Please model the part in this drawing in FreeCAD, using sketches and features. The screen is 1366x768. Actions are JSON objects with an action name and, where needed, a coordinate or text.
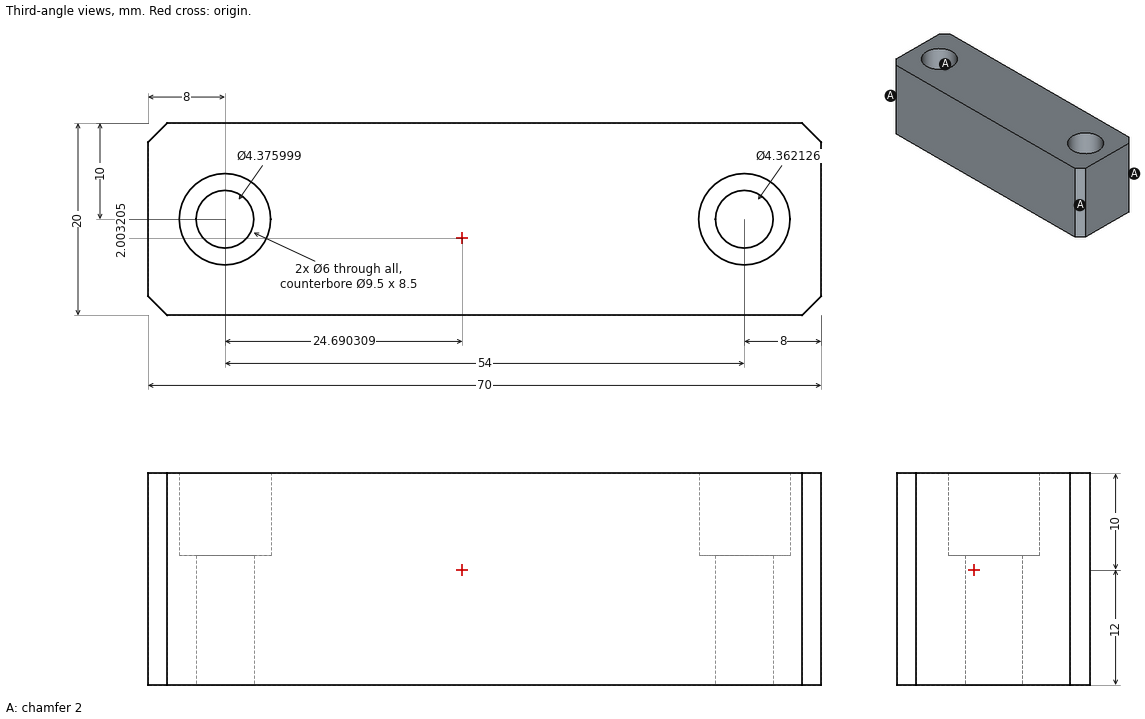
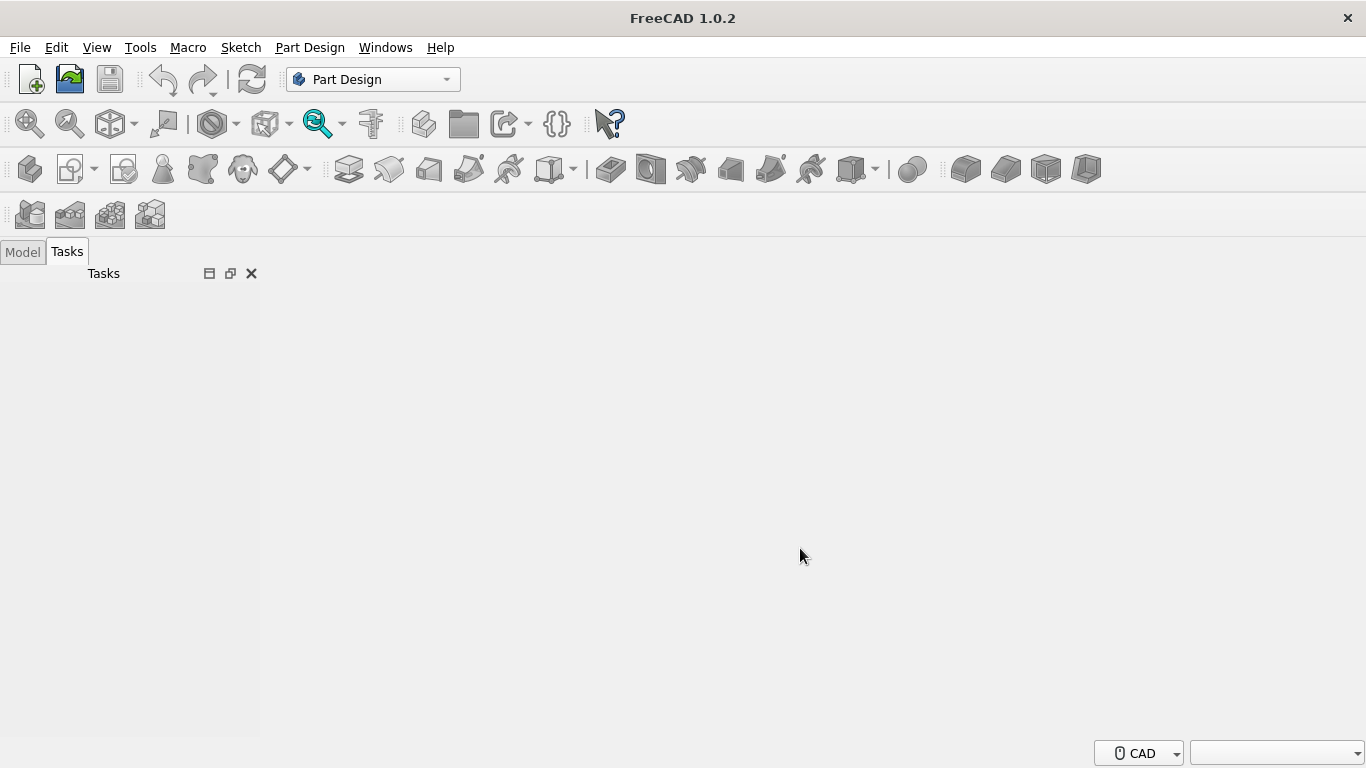
{"action": "left_click", "coordinate": [30, 80]}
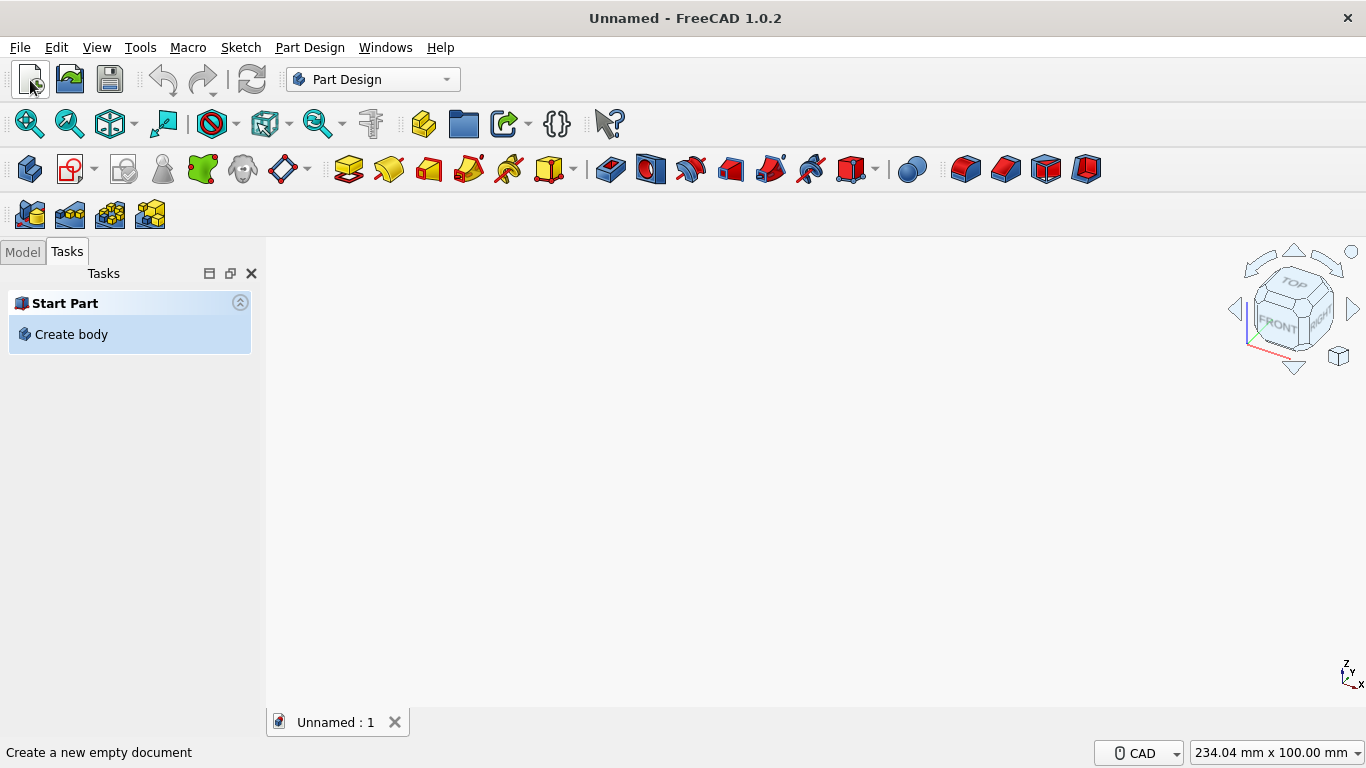
{"action": "left_click", "coordinate": [70, 170]}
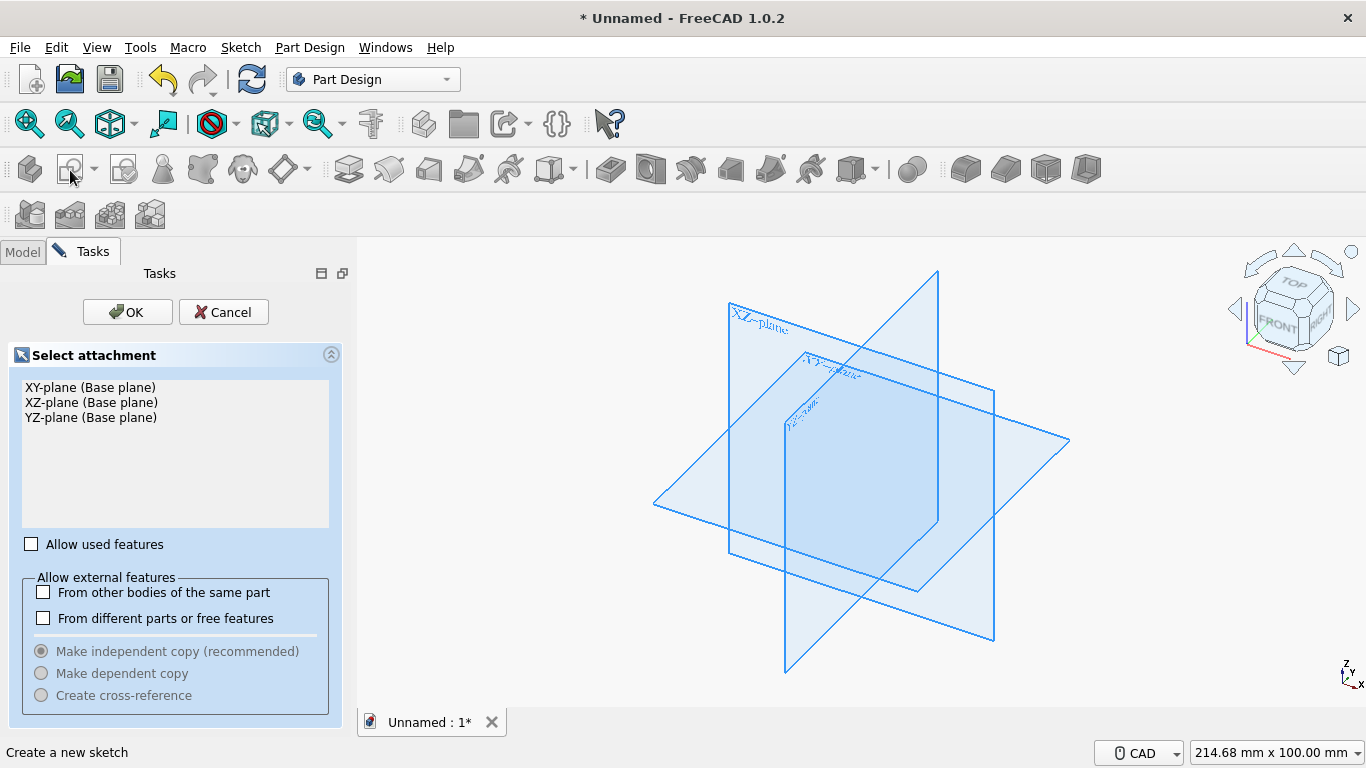
{"action": "left_click", "coordinate": [82, 388]}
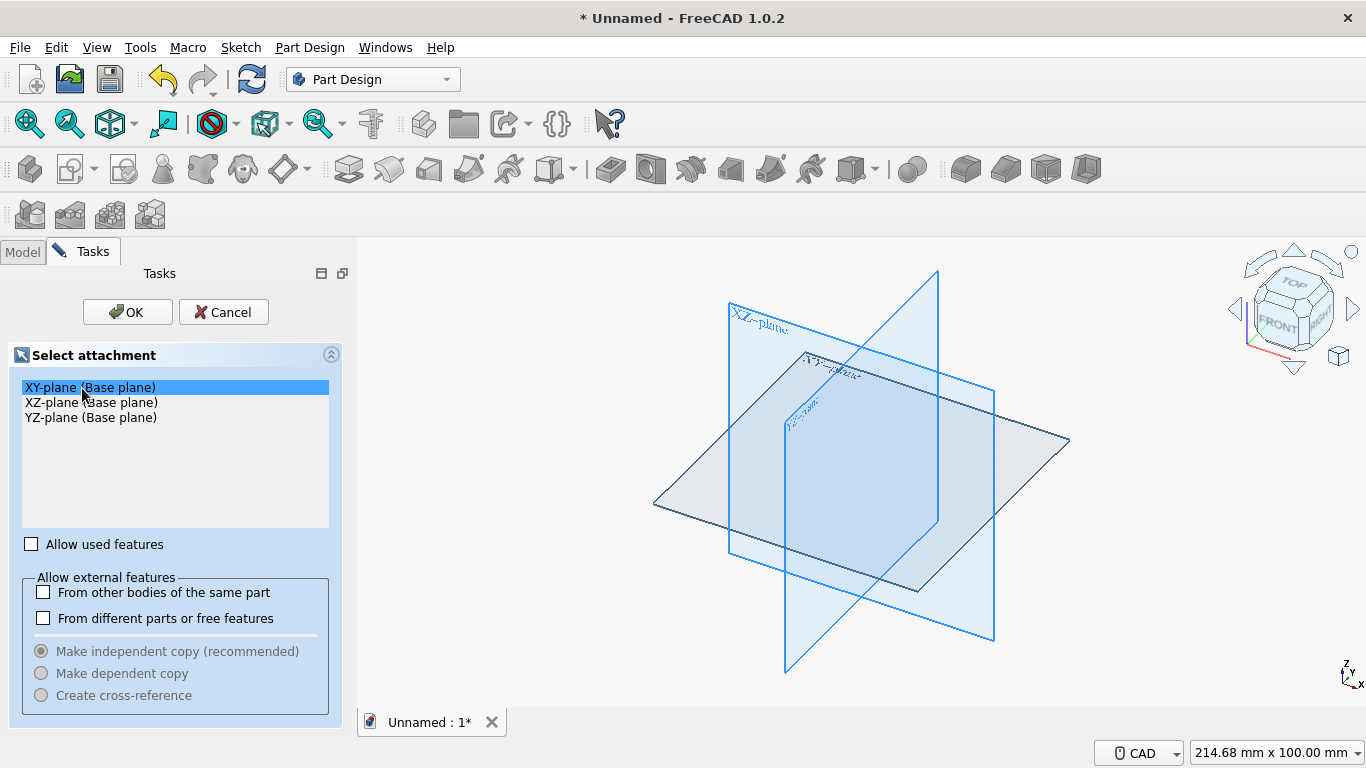
{"action": "left_click", "coordinate": [128, 312]}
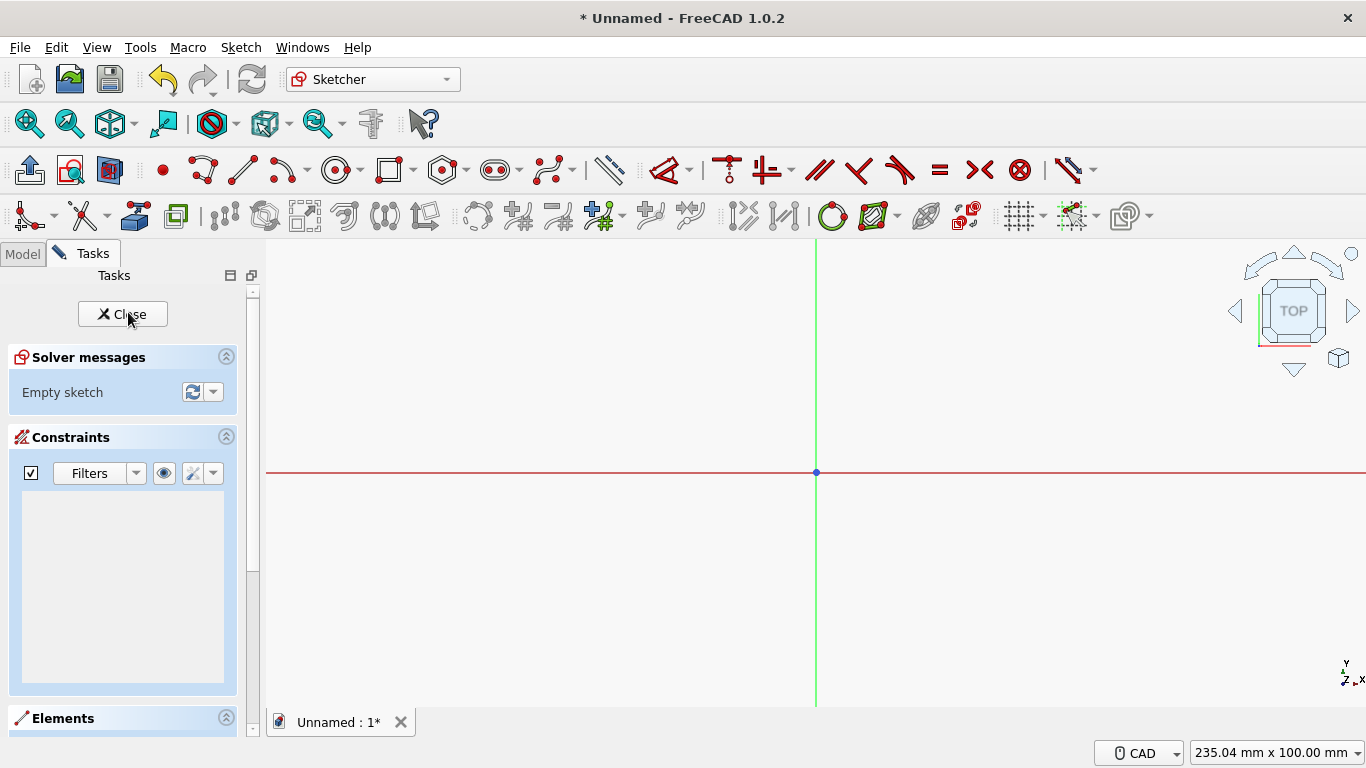
{"action": "scroll", "coordinate": [923, 452], "scroll_direction": "up", "scroll_amount": 3}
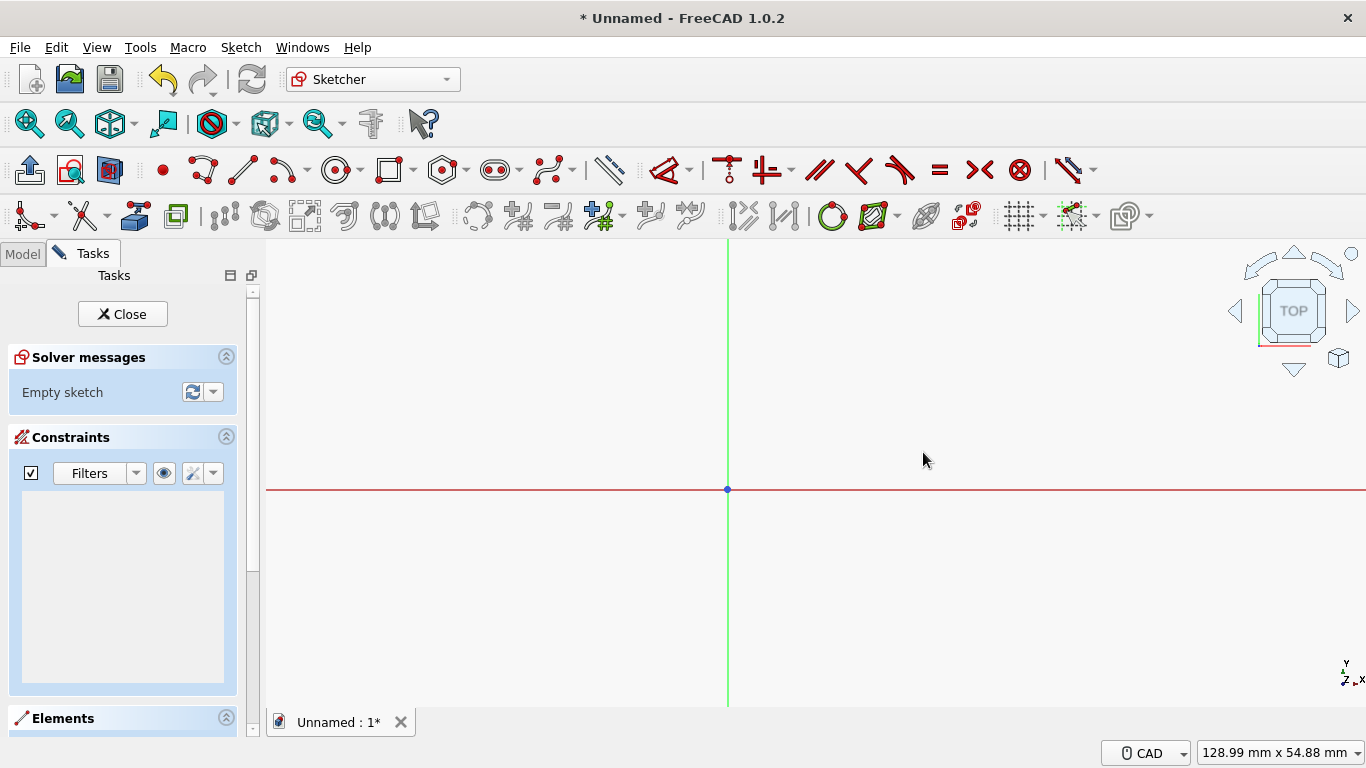
{"action": "left_click", "coordinate": [390, 170]}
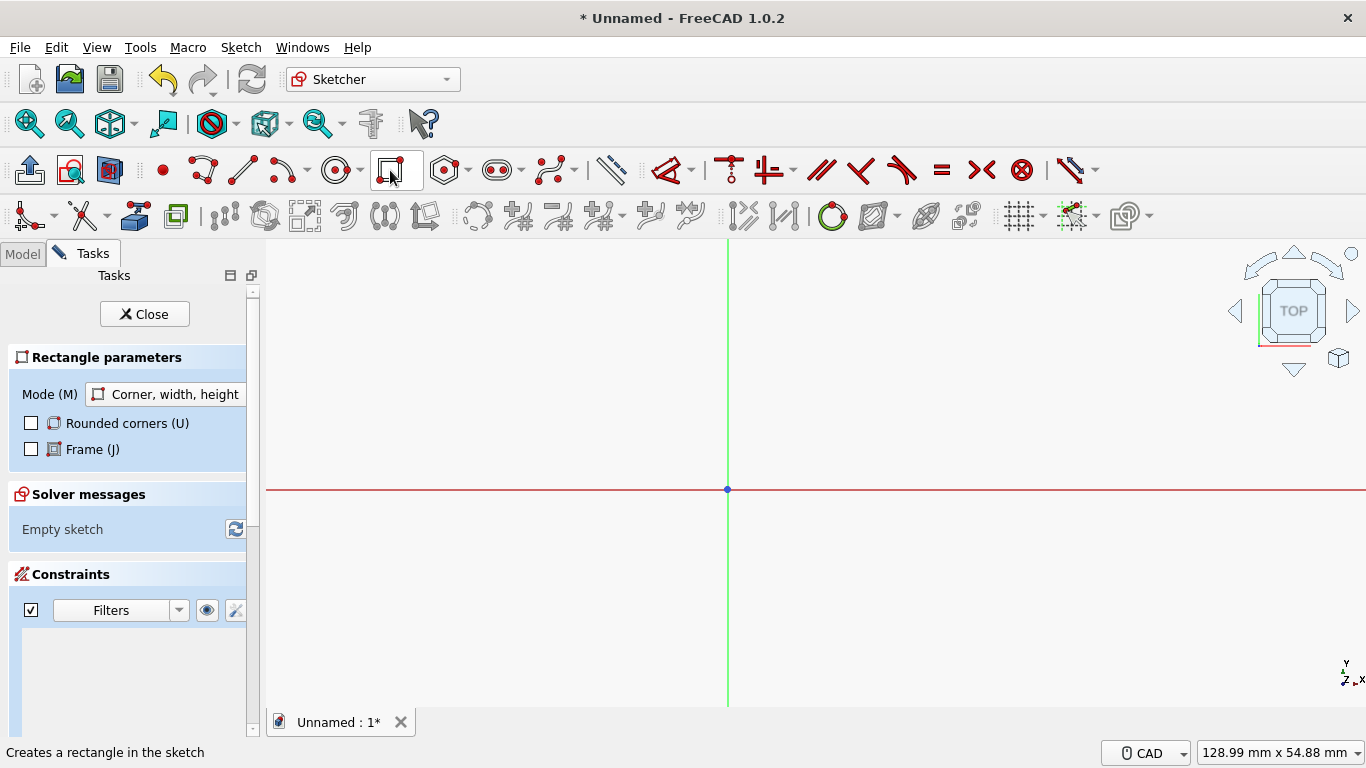
{"action": "left_click", "coordinate": [449, 388]}
{"action": "left_click", "coordinate": [1046, 558]}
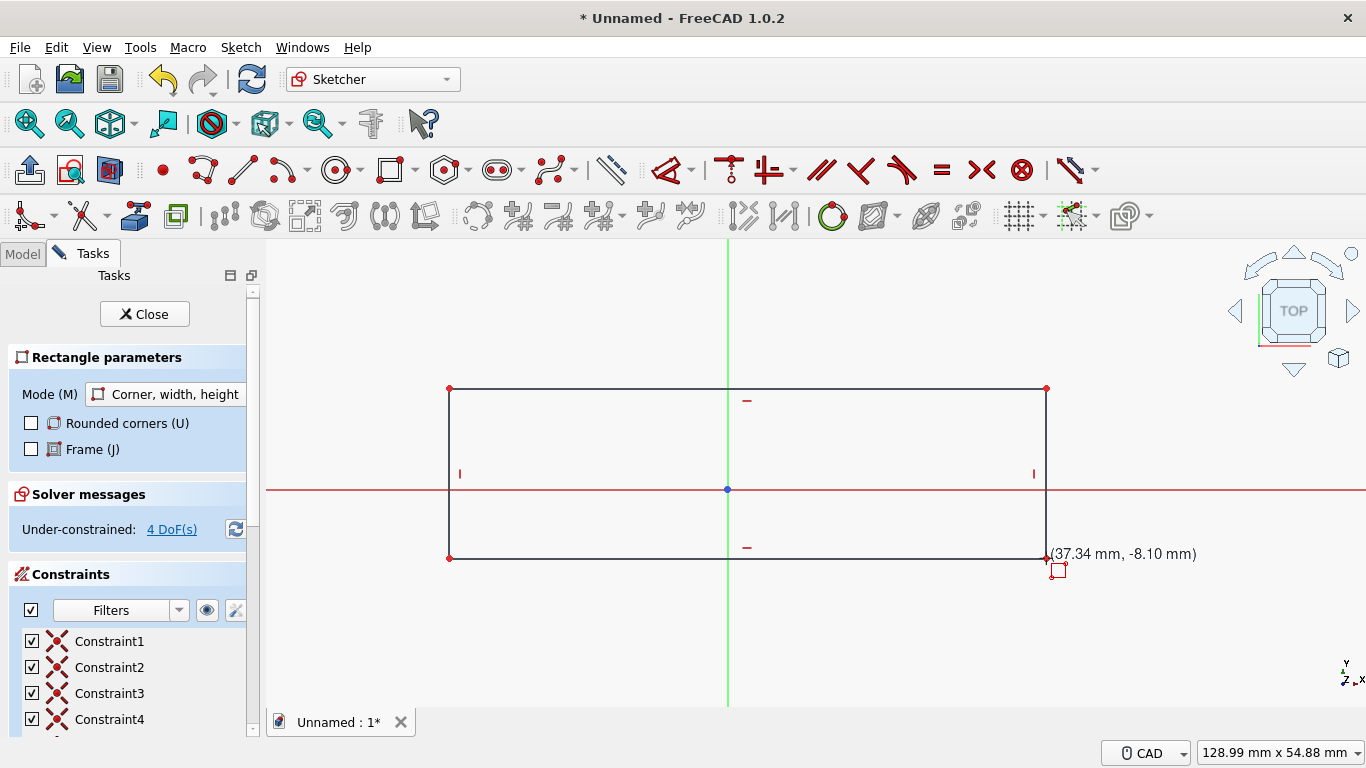
{"action": "key", "text": "g c"}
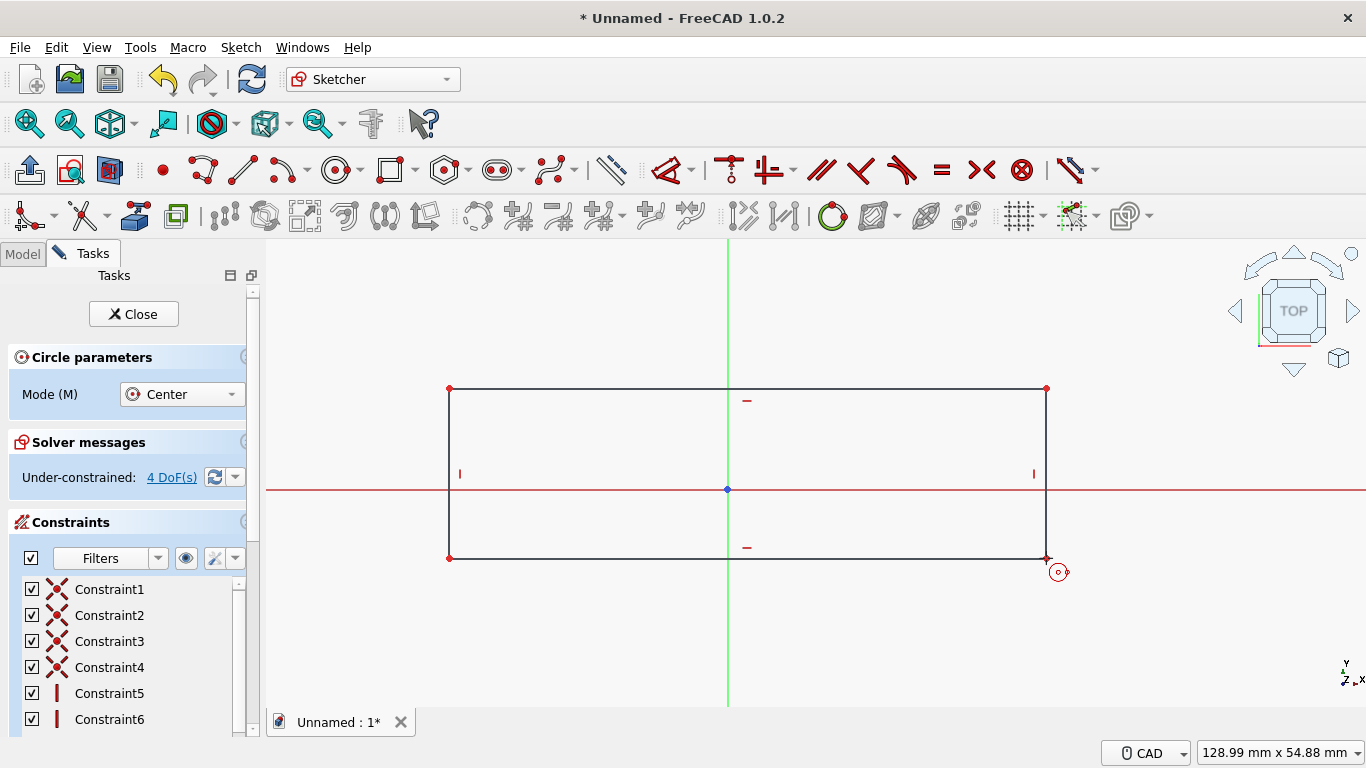
{"action": "left_click", "coordinate": [517, 473]}
{"action": "left_click", "coordinate": [530, 460]}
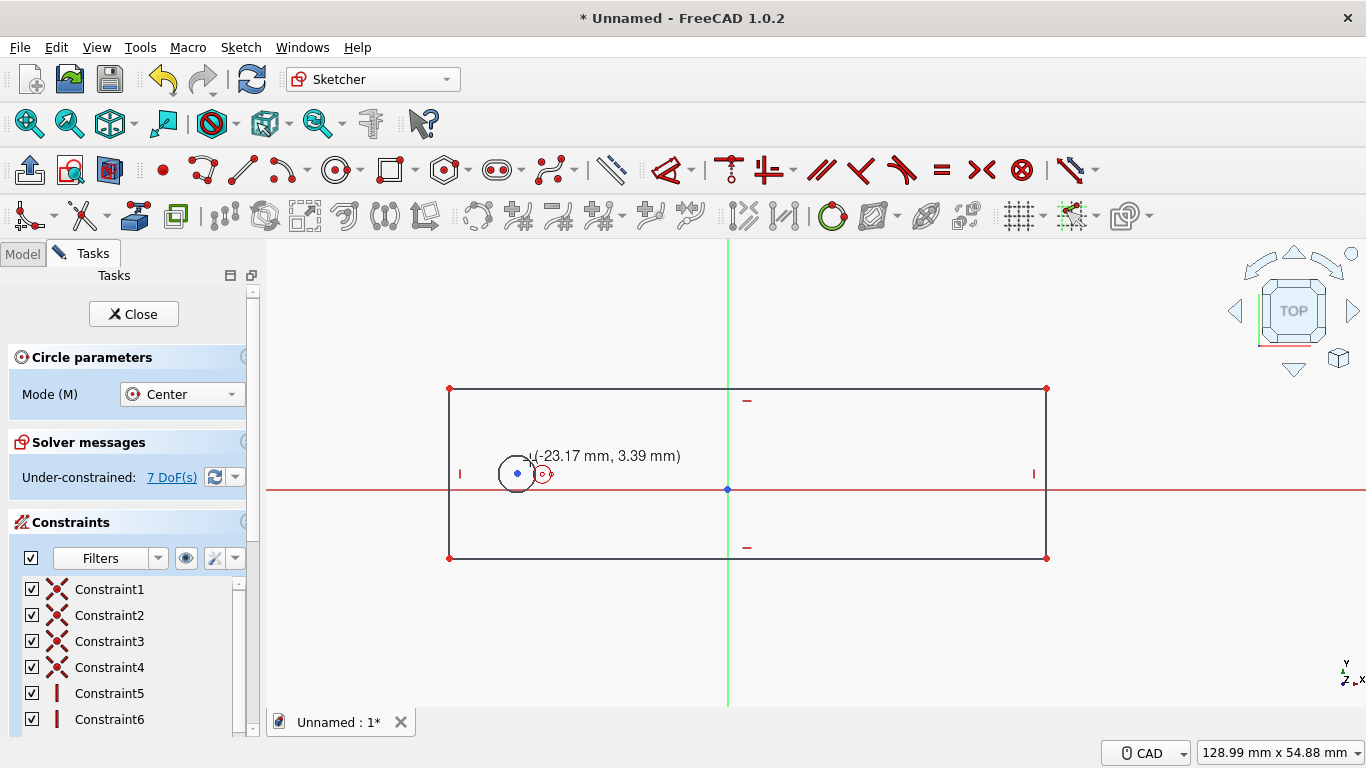
{"action": "left_click", "coordinate": [977, 473]}
{"action": "left_click", "coordinate": [991, 460]}
{"action": "key", "text": "Escape"}